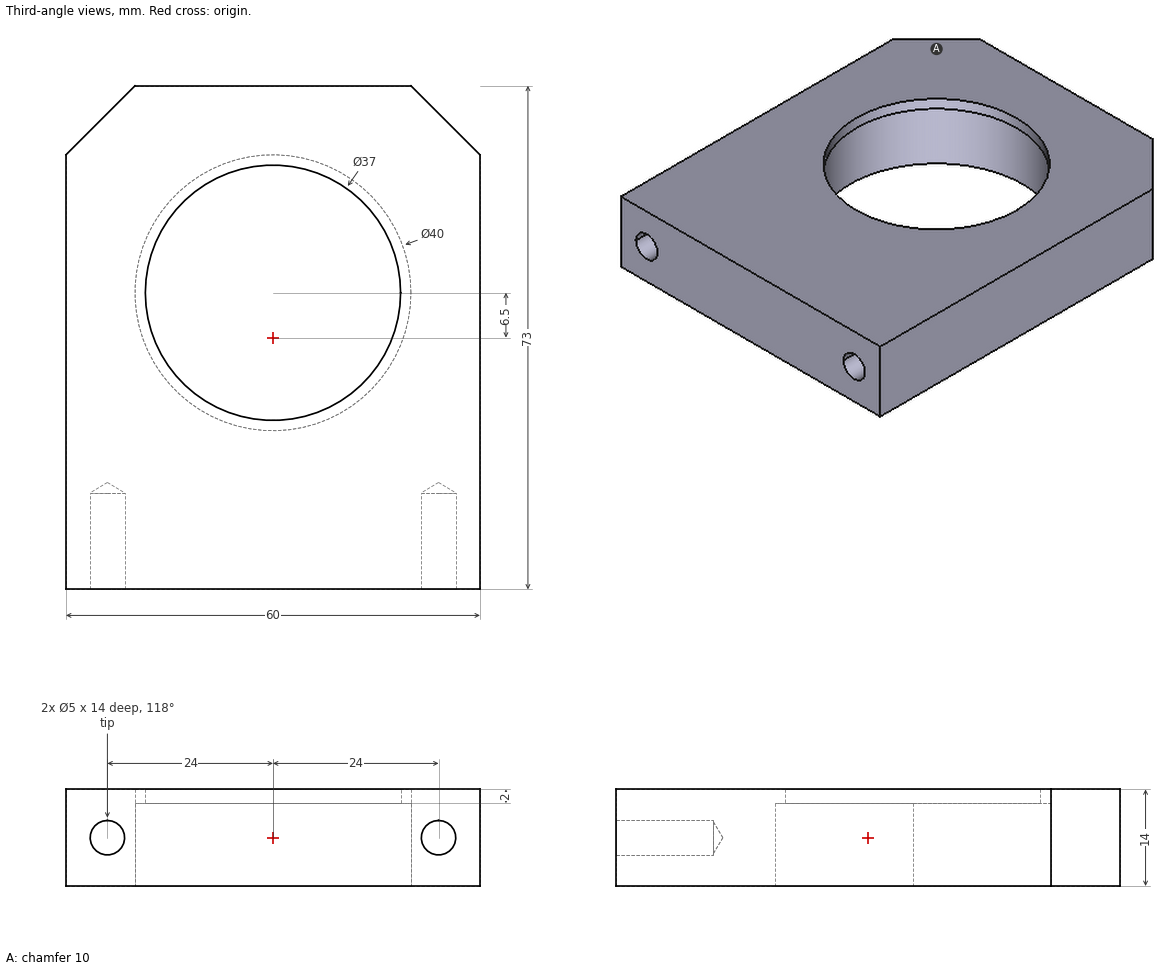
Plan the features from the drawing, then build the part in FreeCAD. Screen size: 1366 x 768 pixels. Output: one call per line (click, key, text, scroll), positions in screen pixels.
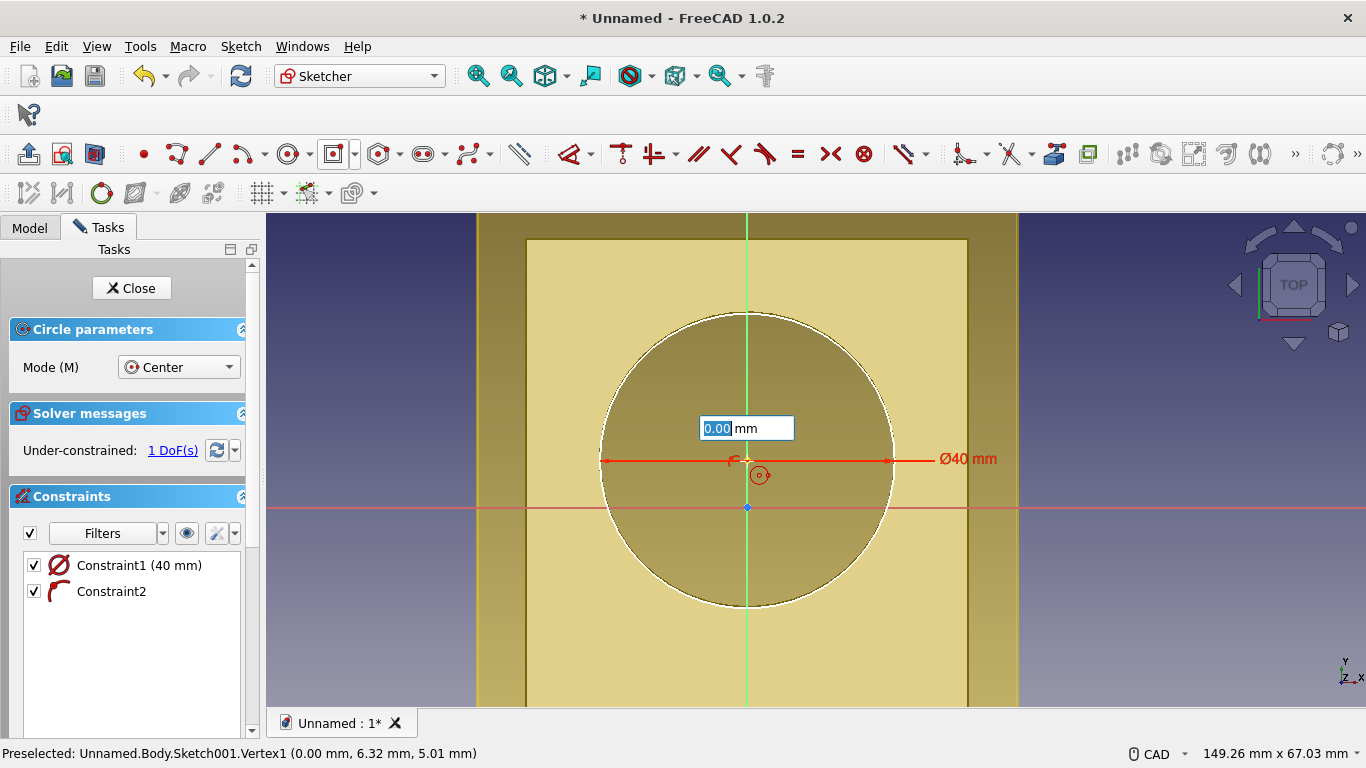
scroll(844, 363, up, 2)
move(843, 363)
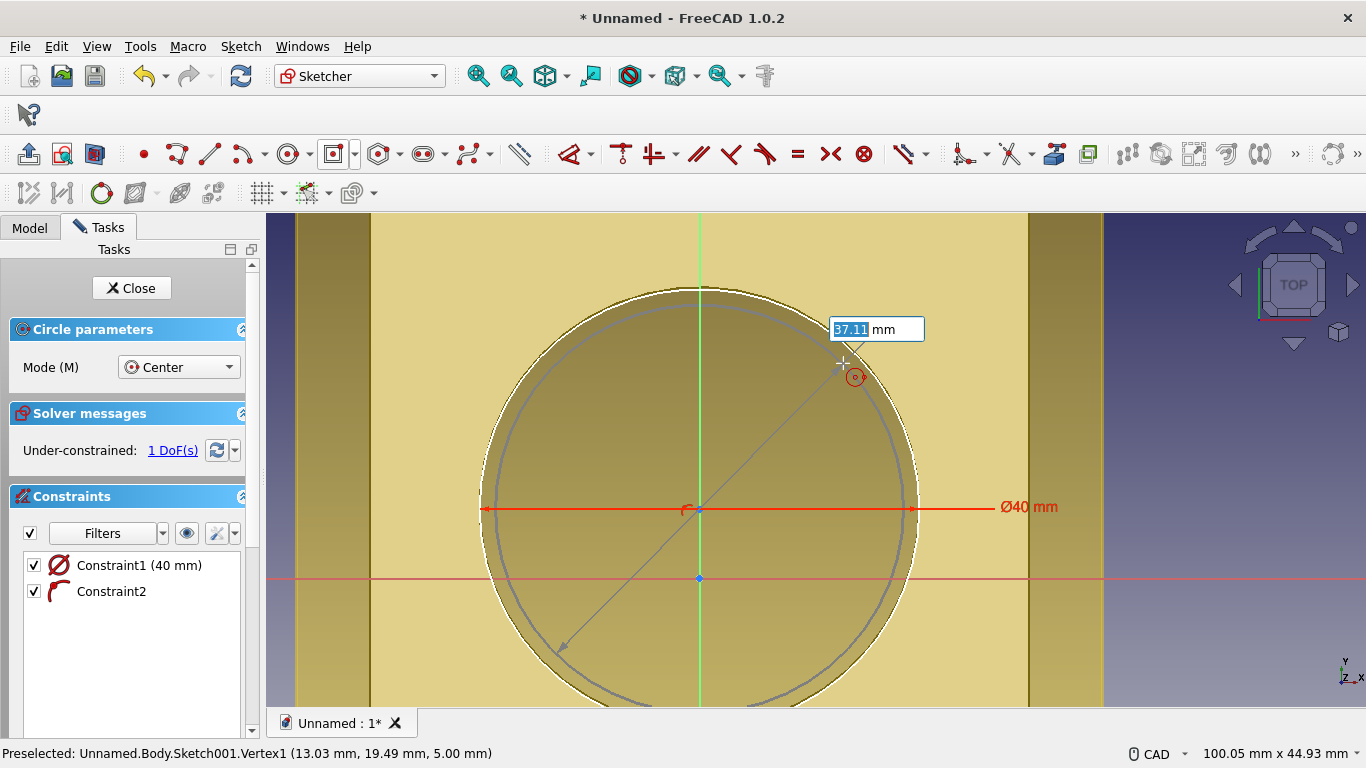
text(37)
key(Return)
key(Escape)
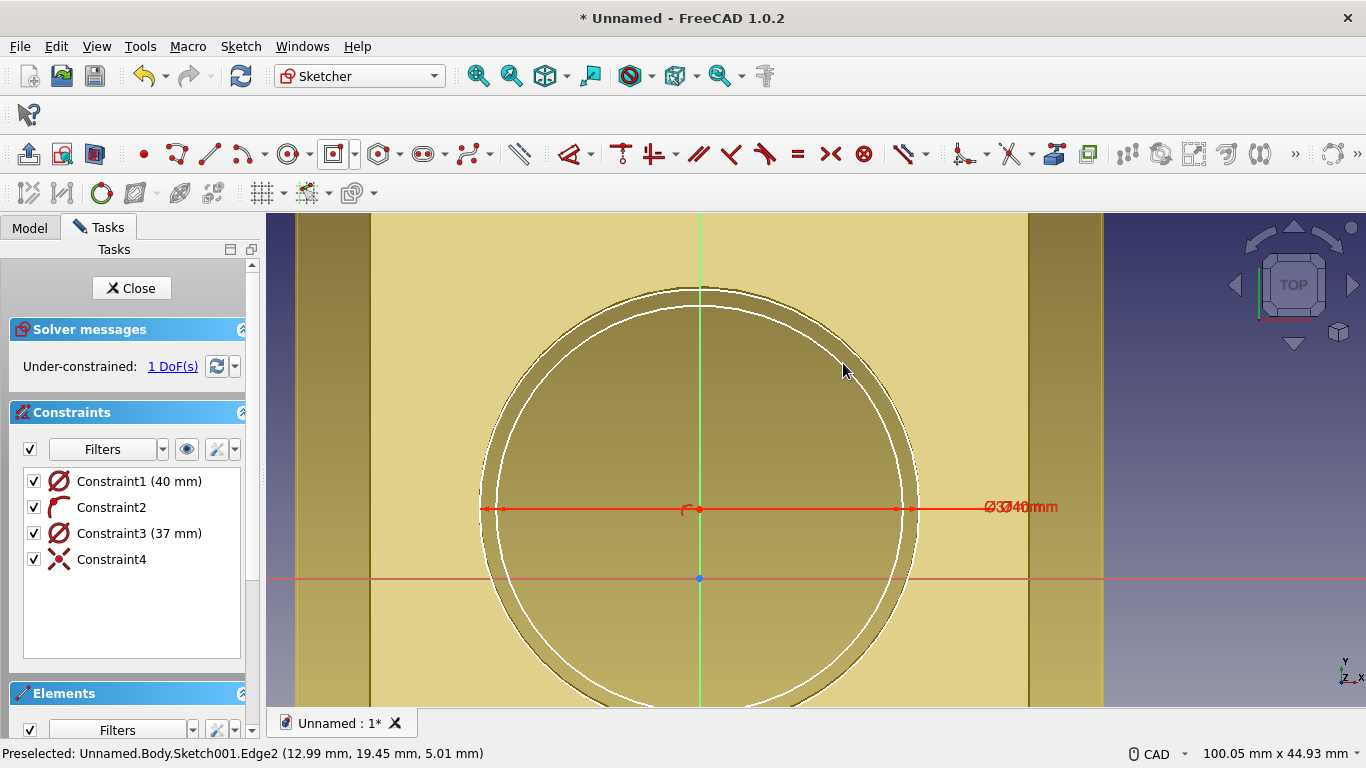
click(568, 154)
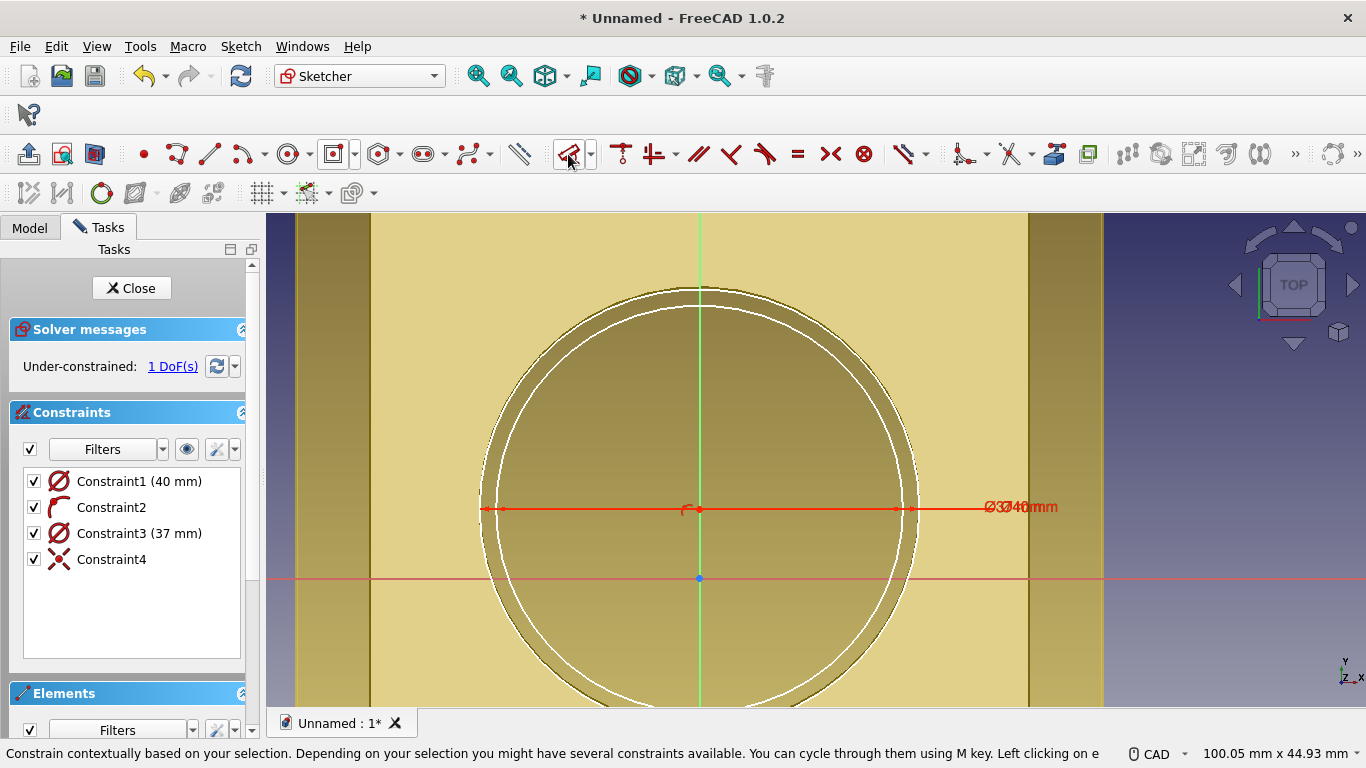
click(700, 509)
click(734, 544)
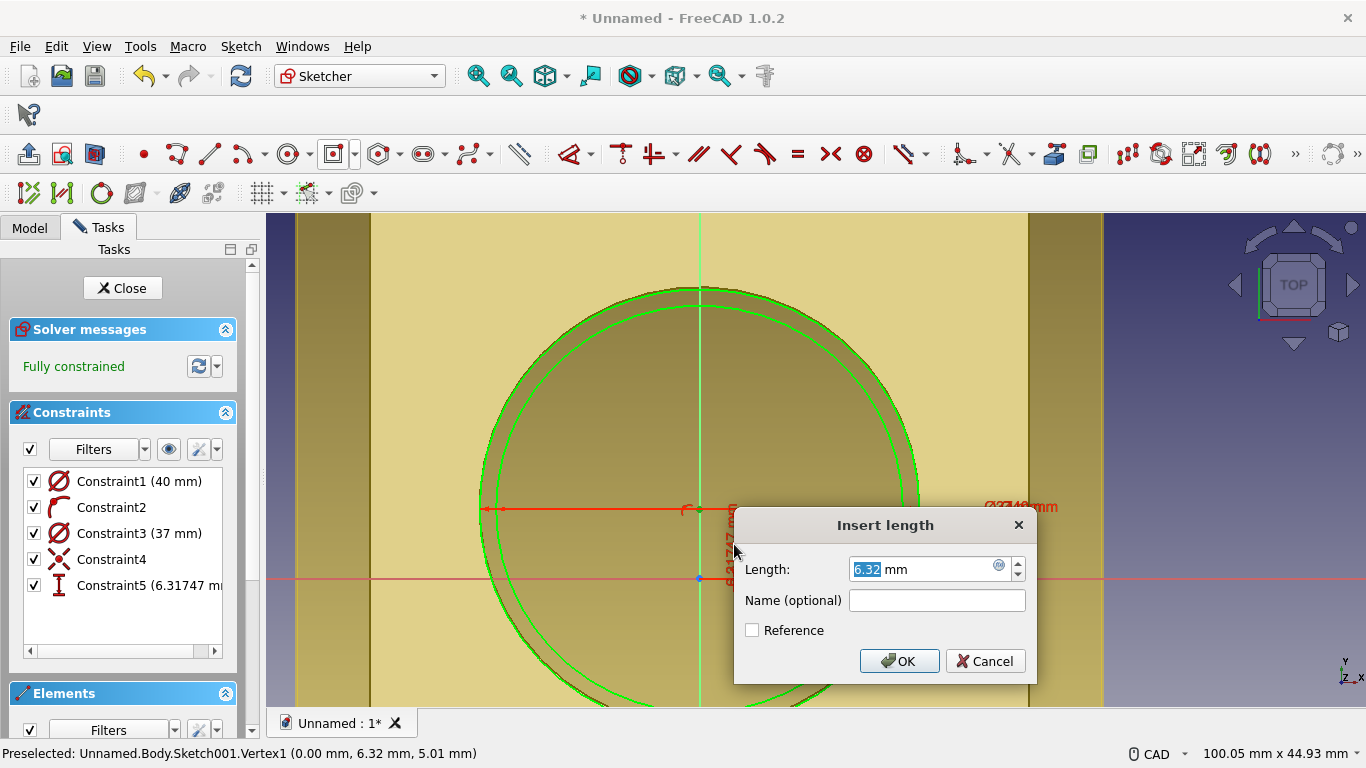
text(6.5)
key(Return)
key(Escape)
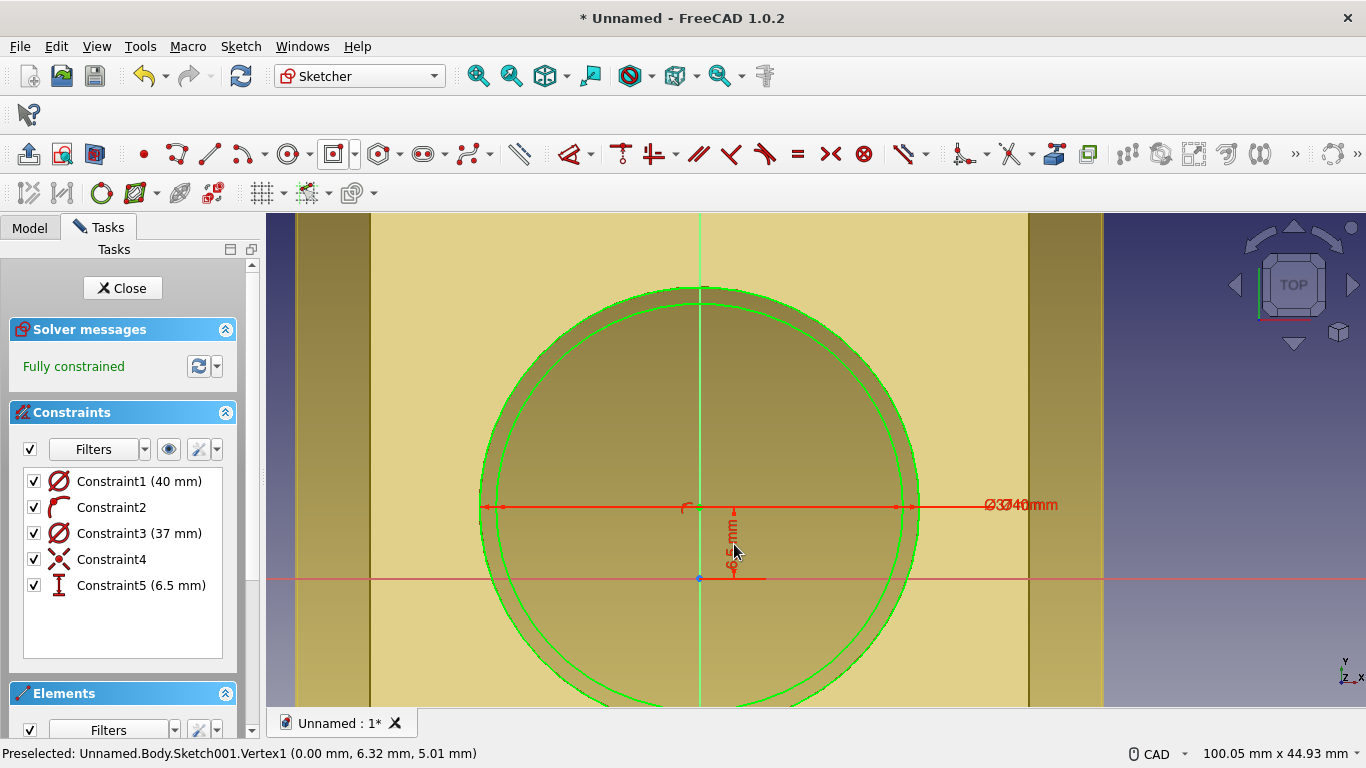
click(123, 288)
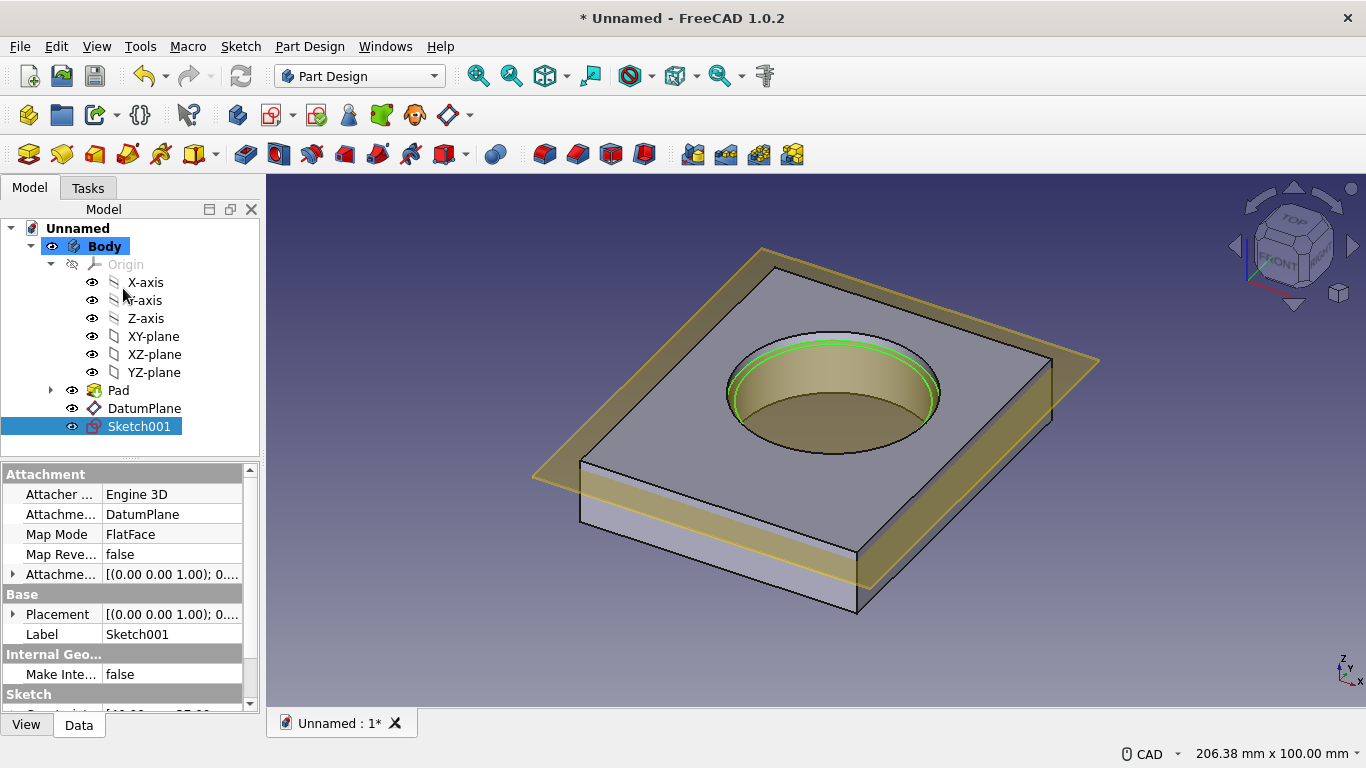
click(29, 154)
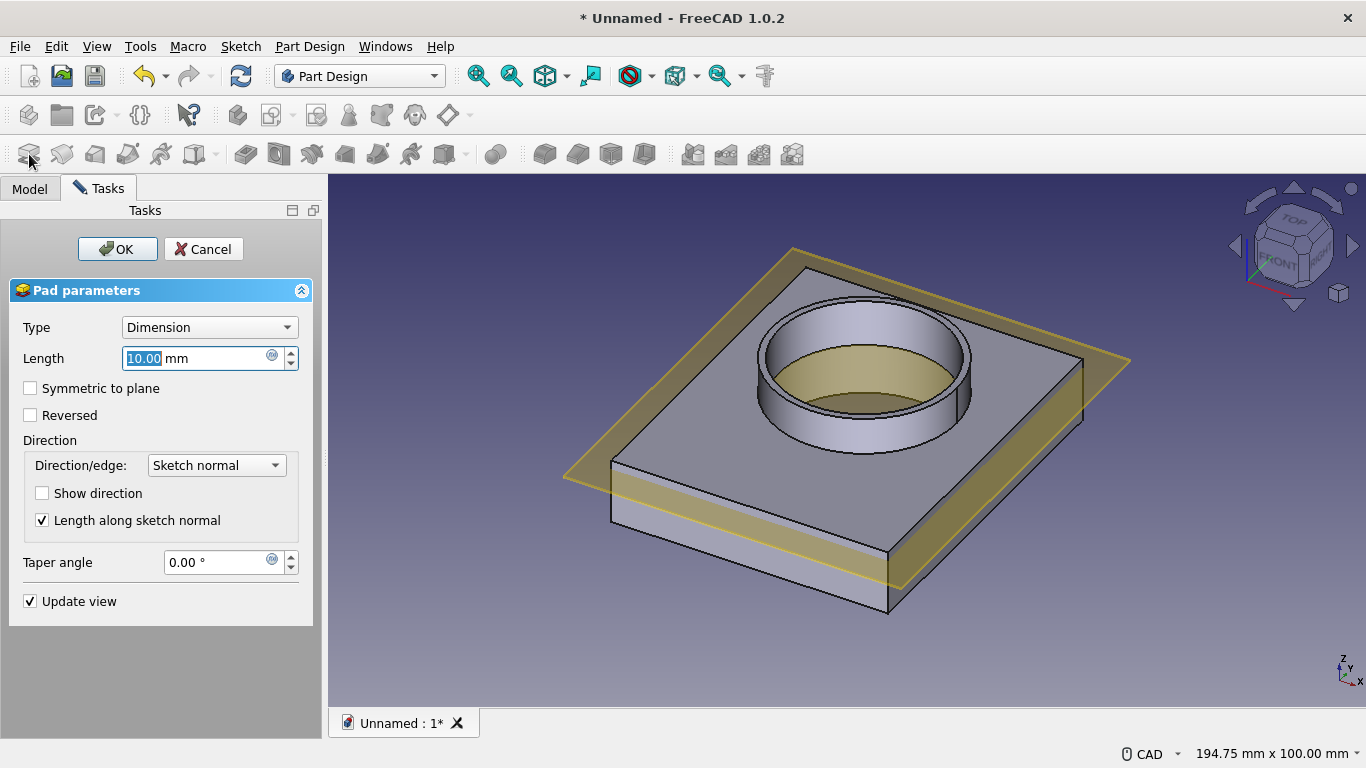
text(2)
key(Tab)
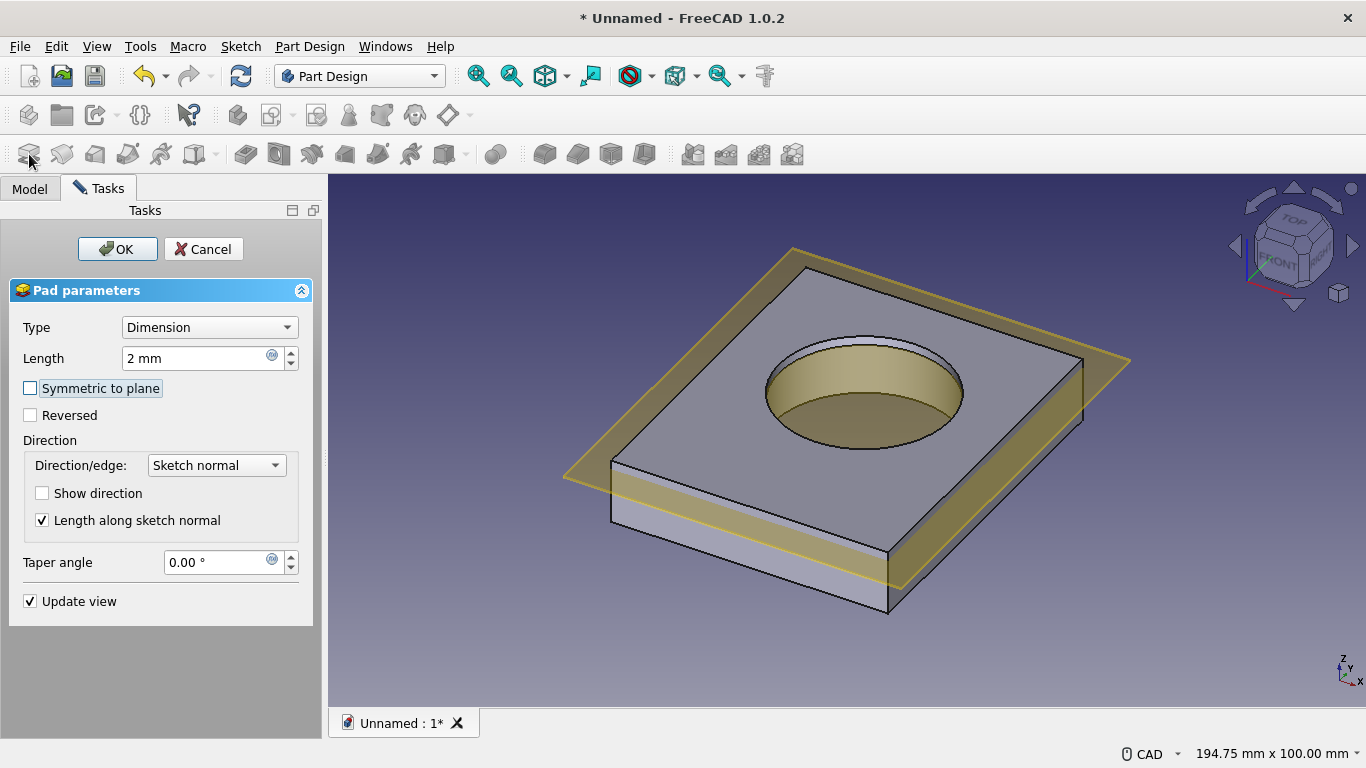
click(118, 249)